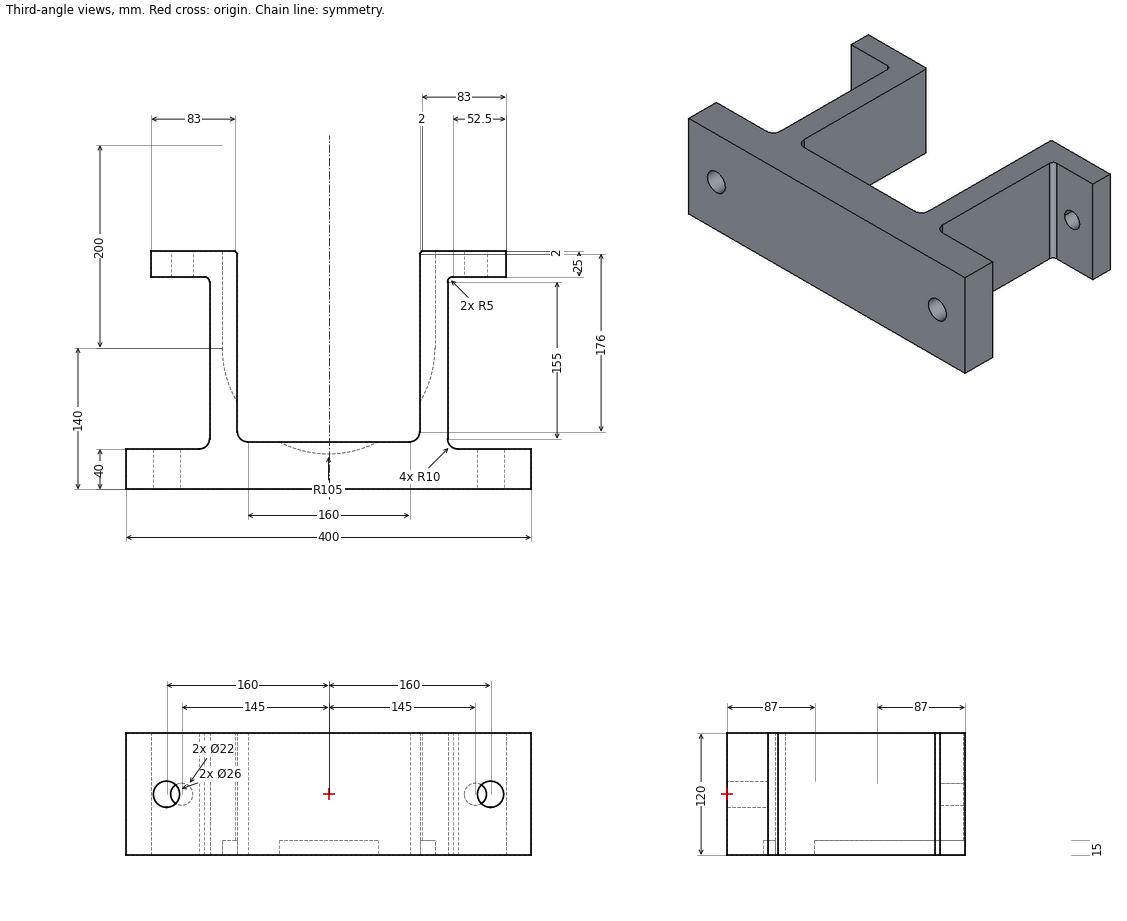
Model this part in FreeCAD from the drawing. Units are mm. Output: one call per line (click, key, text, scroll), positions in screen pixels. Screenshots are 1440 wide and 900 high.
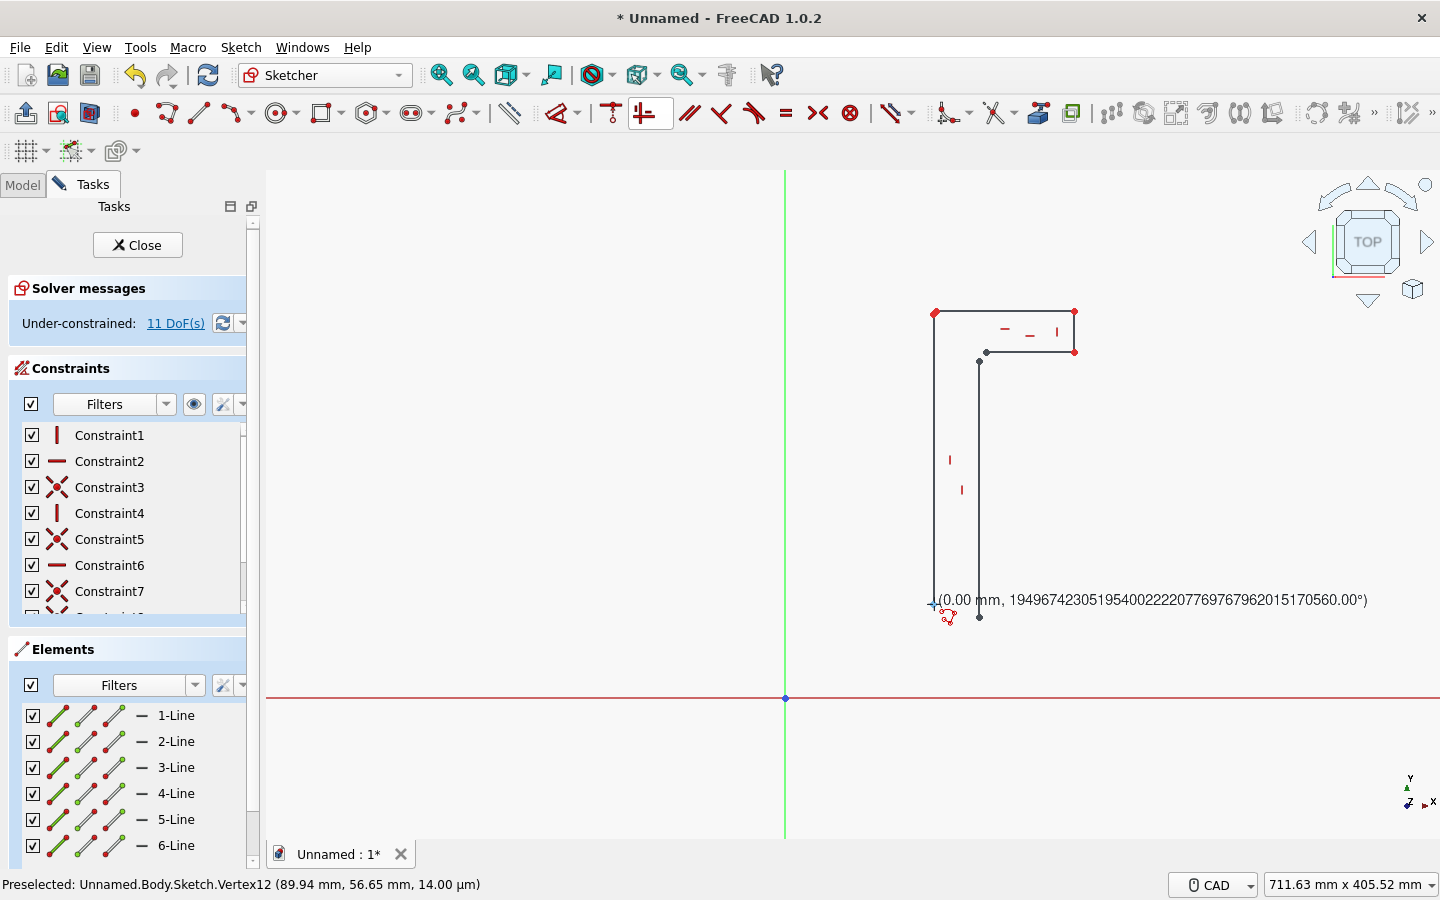
click(200, 114)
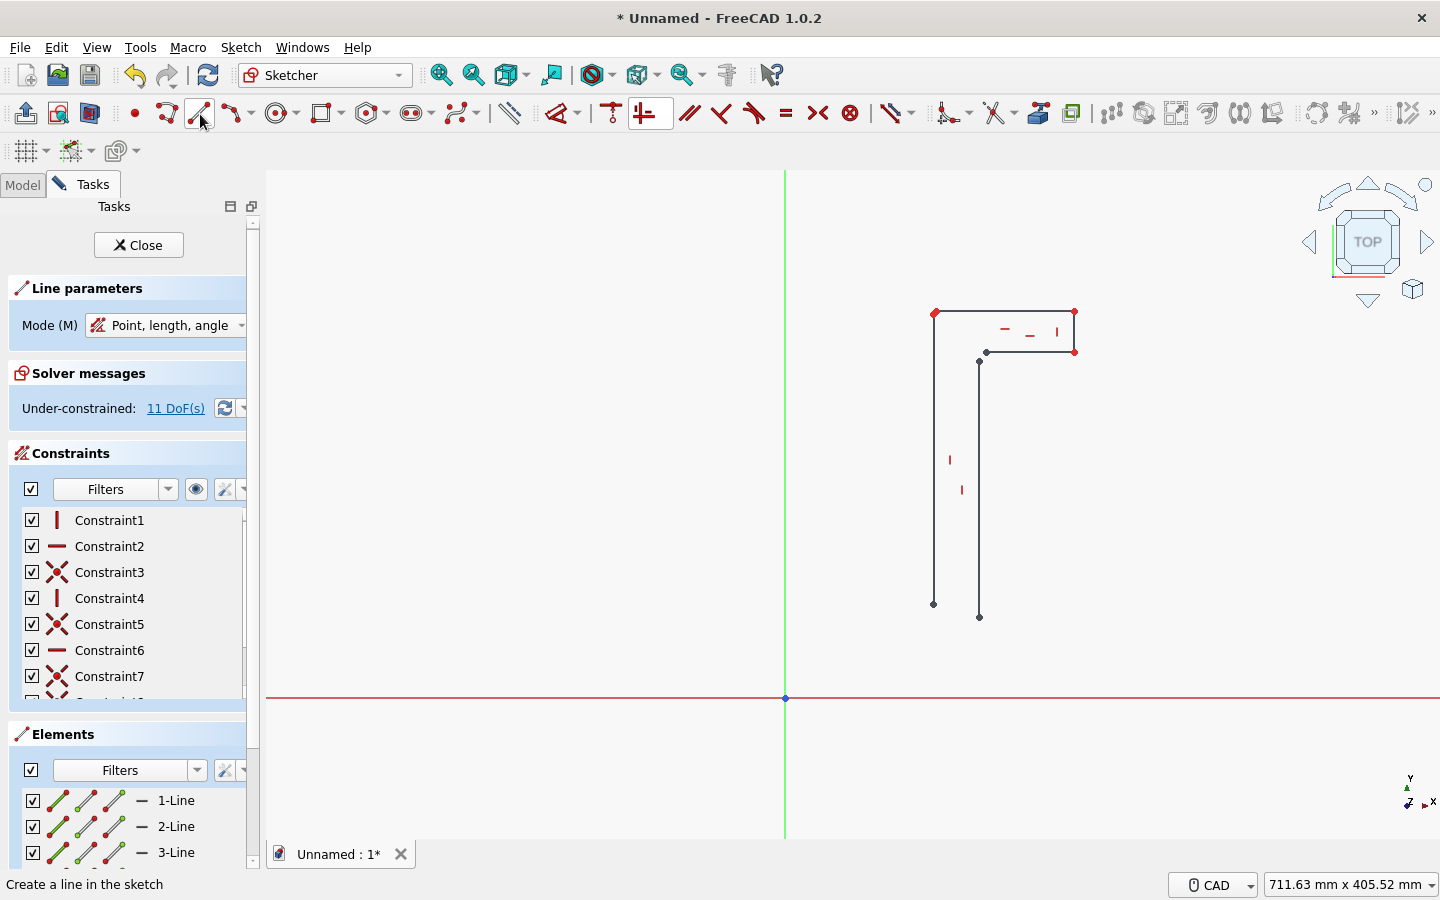
click(917, 621)
click(653, 621)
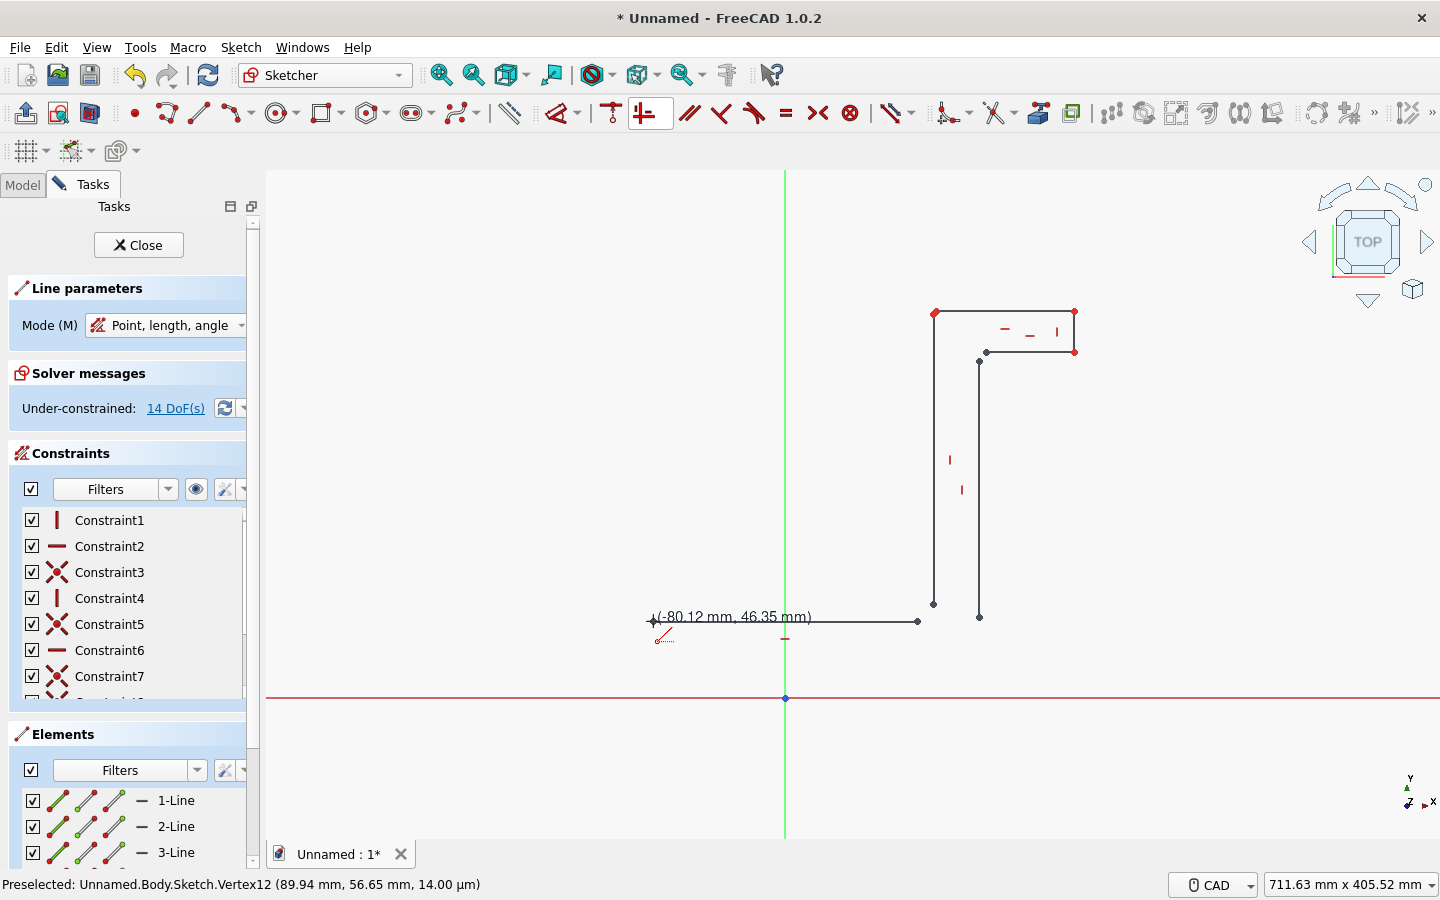
key(g)
key(m)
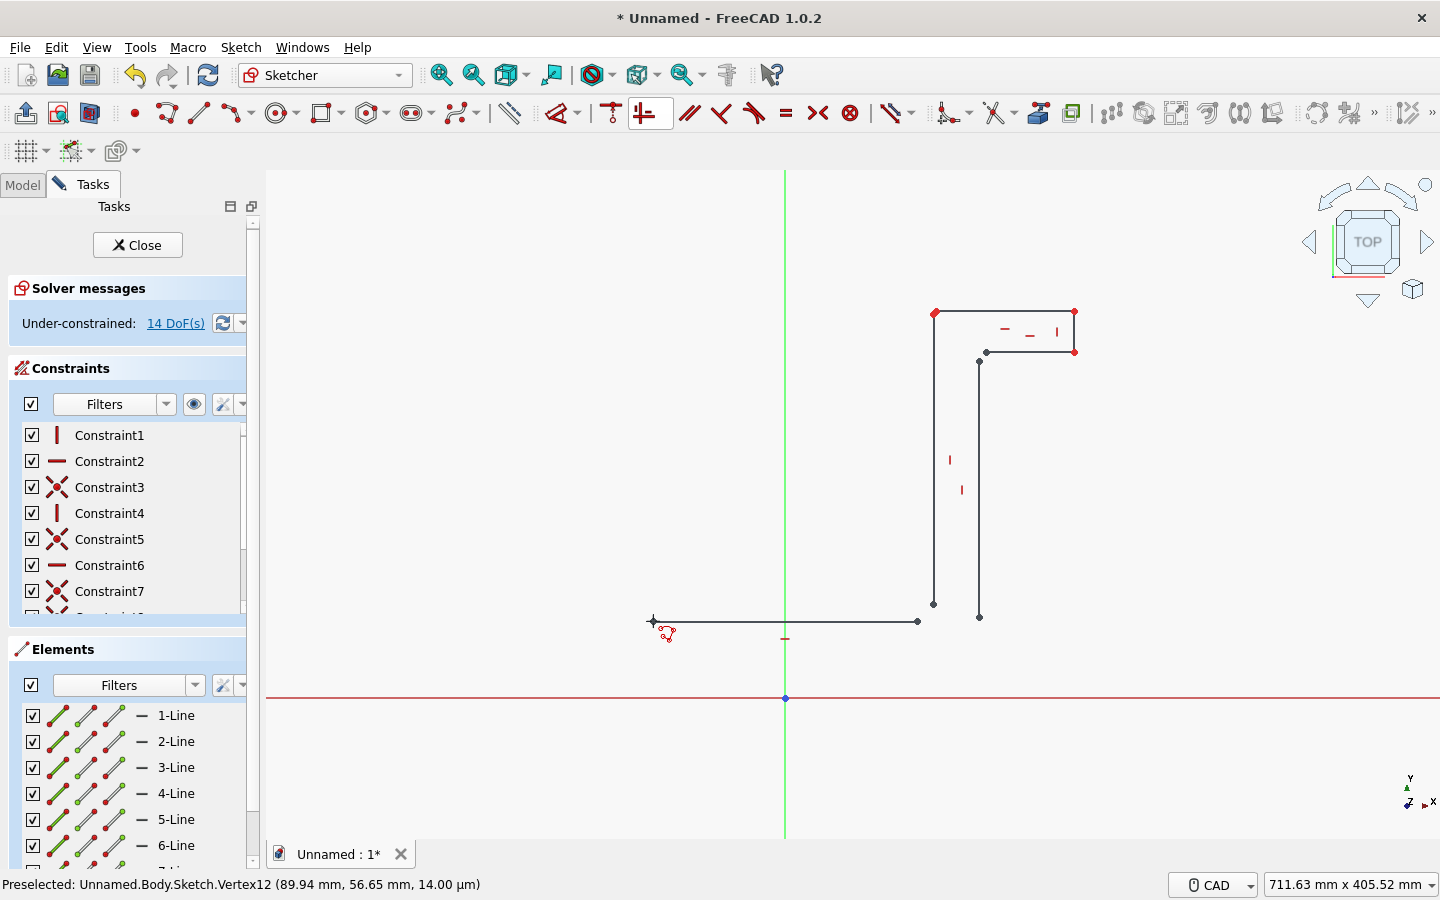
click(637, 604)
click(637, 314)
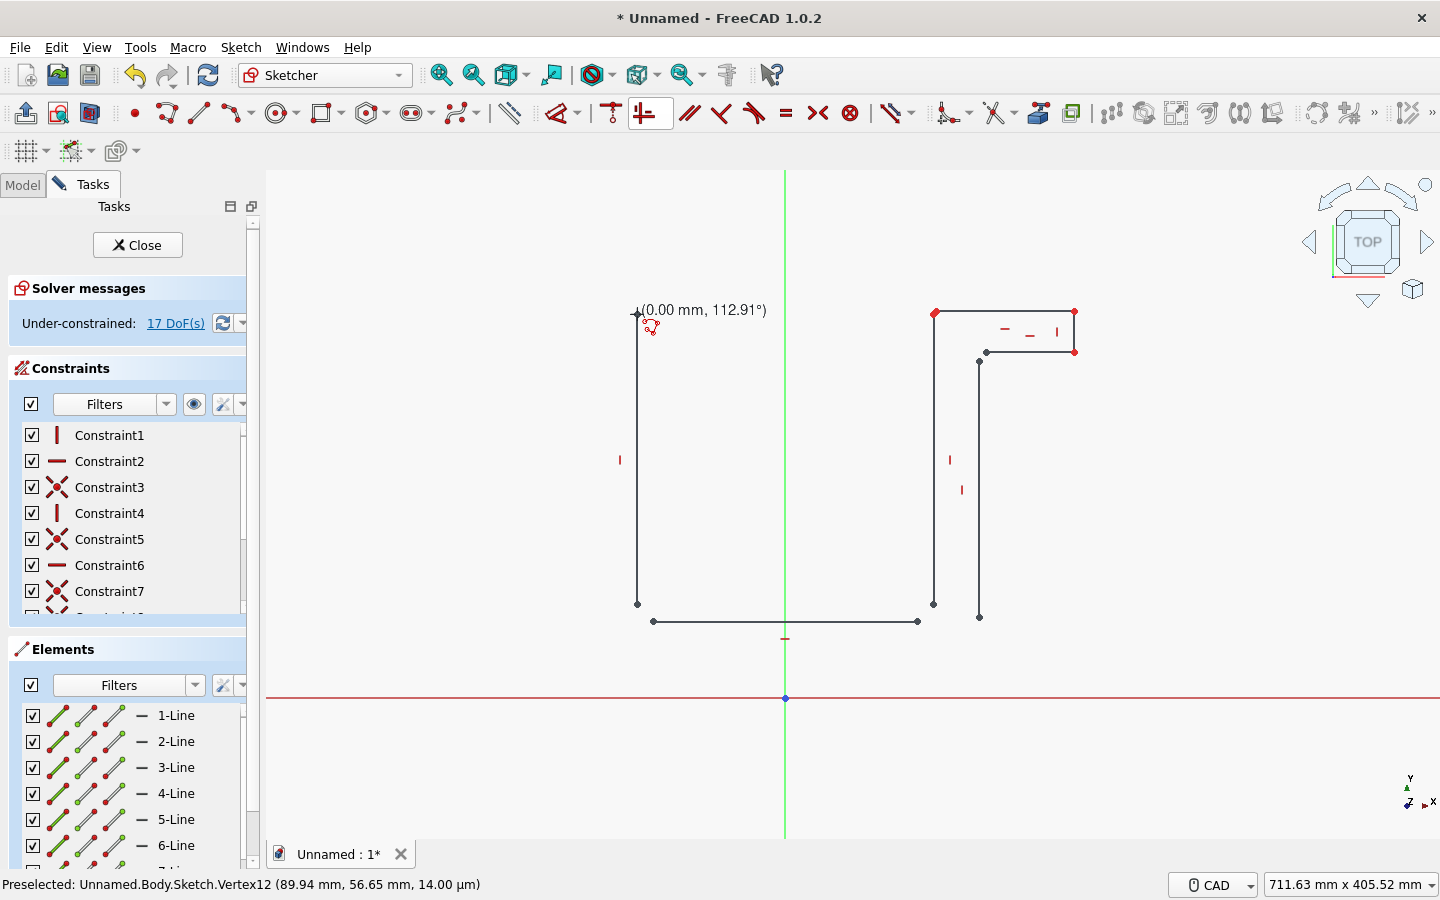
scroll(633, 311, up, 7)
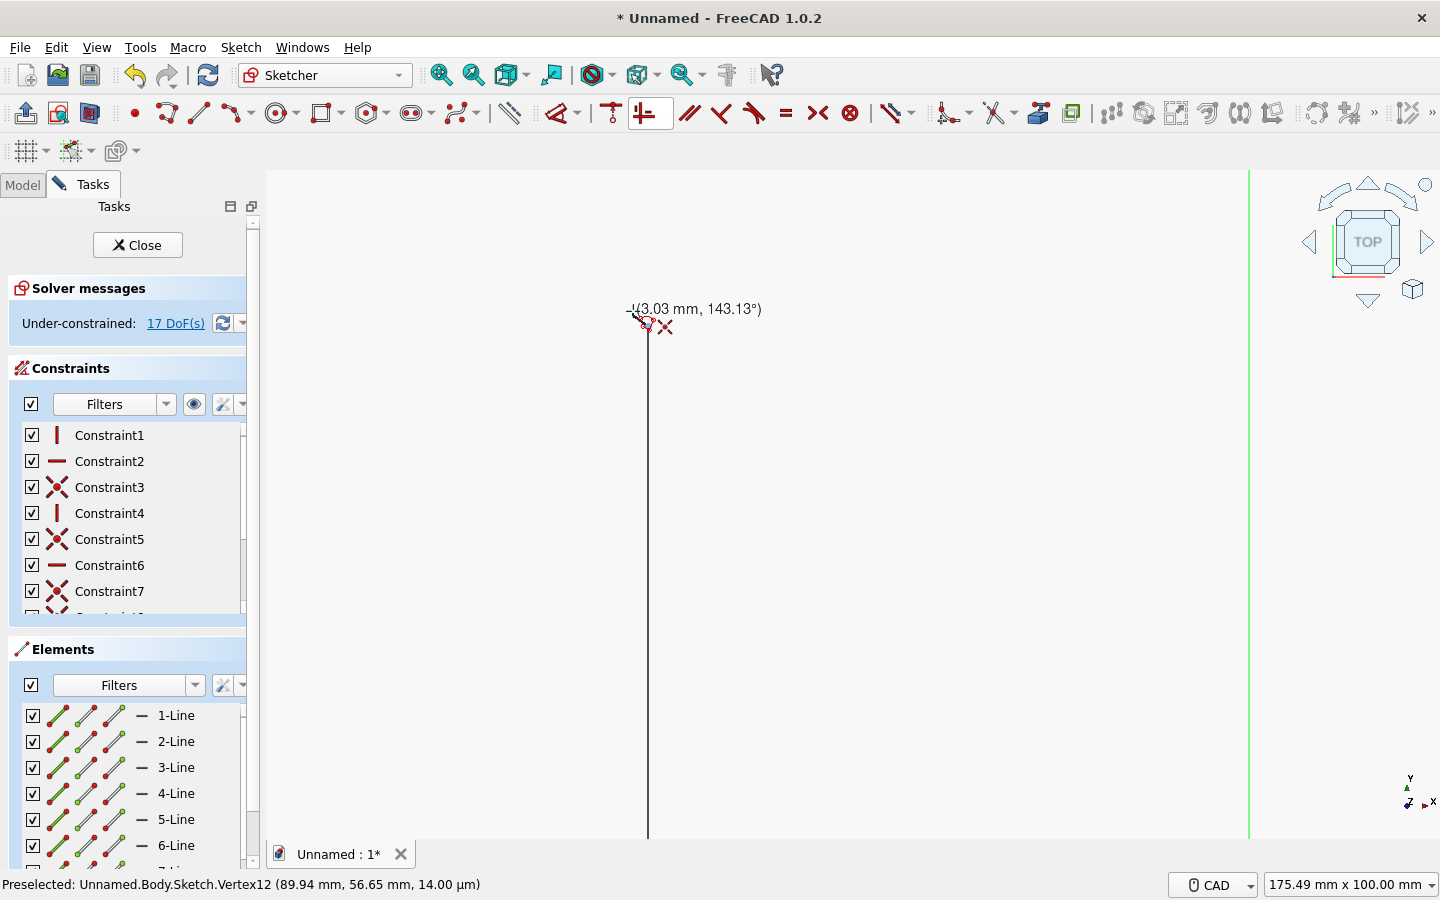
click(634, 309)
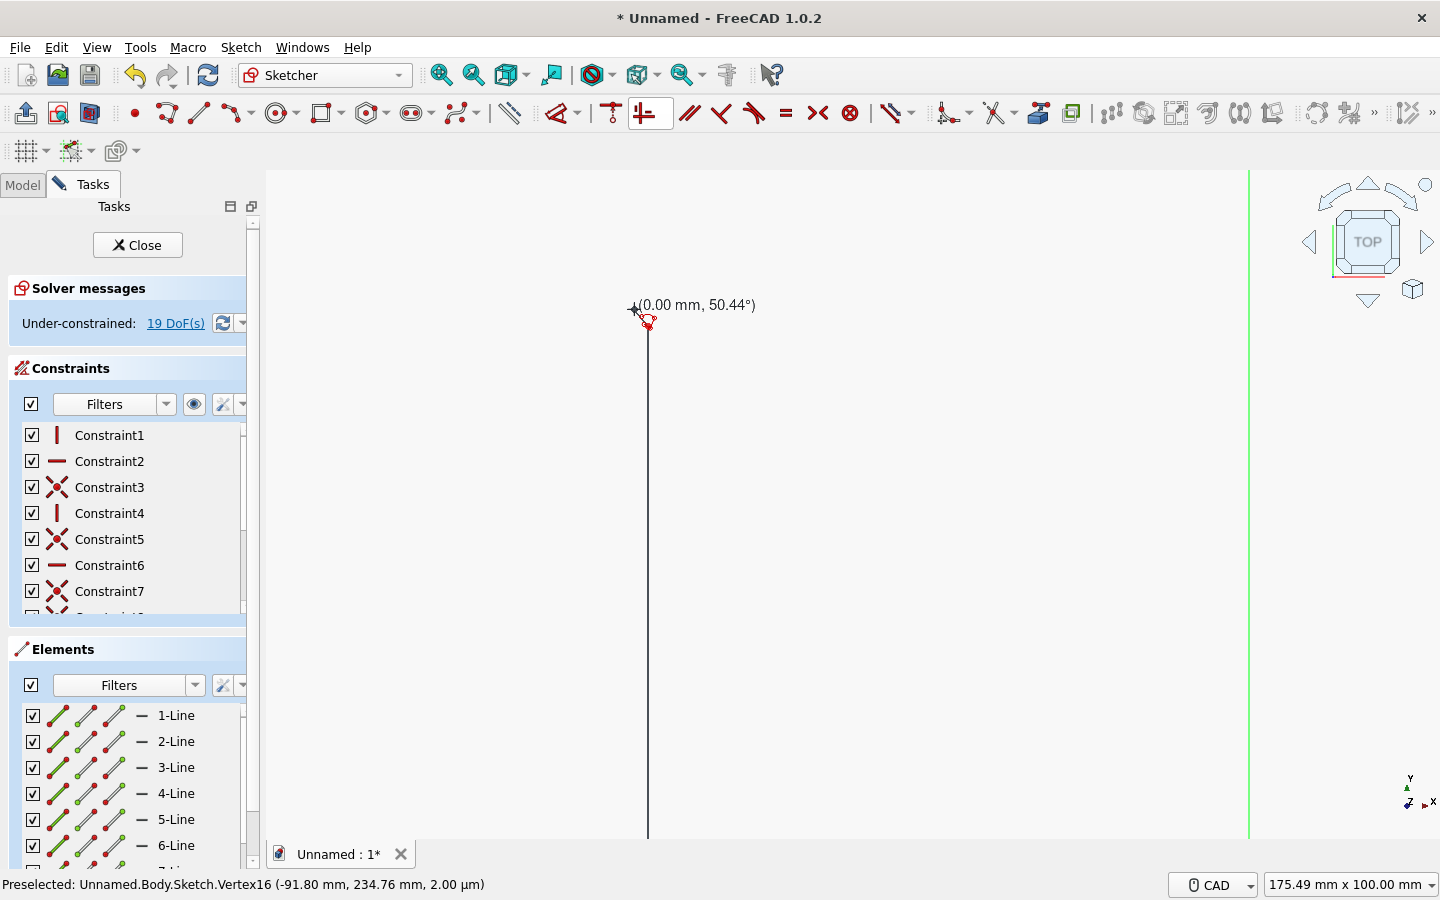
scroll(632, 311, down, 7)